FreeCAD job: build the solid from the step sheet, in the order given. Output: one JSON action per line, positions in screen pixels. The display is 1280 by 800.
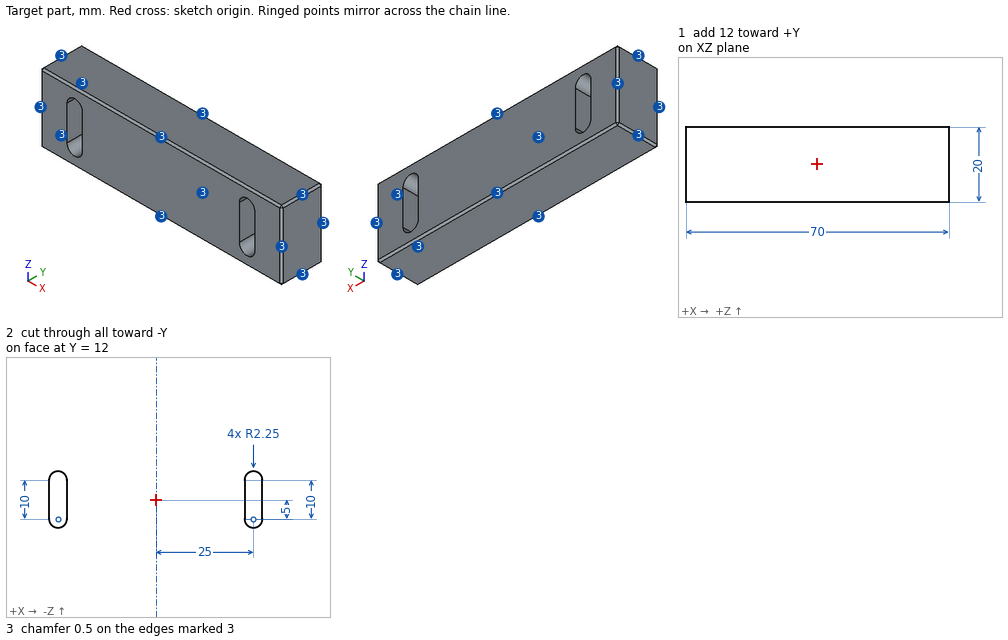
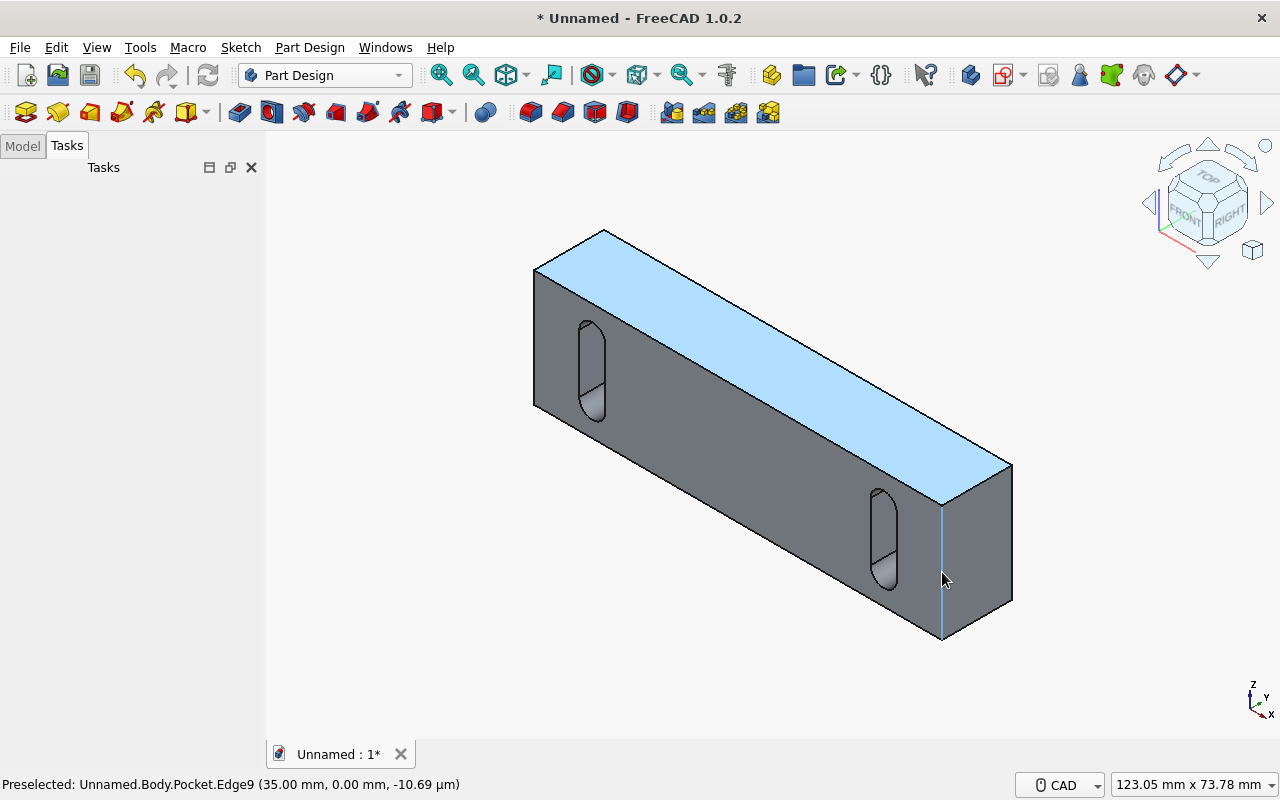
{"action": "key", "text": "2"}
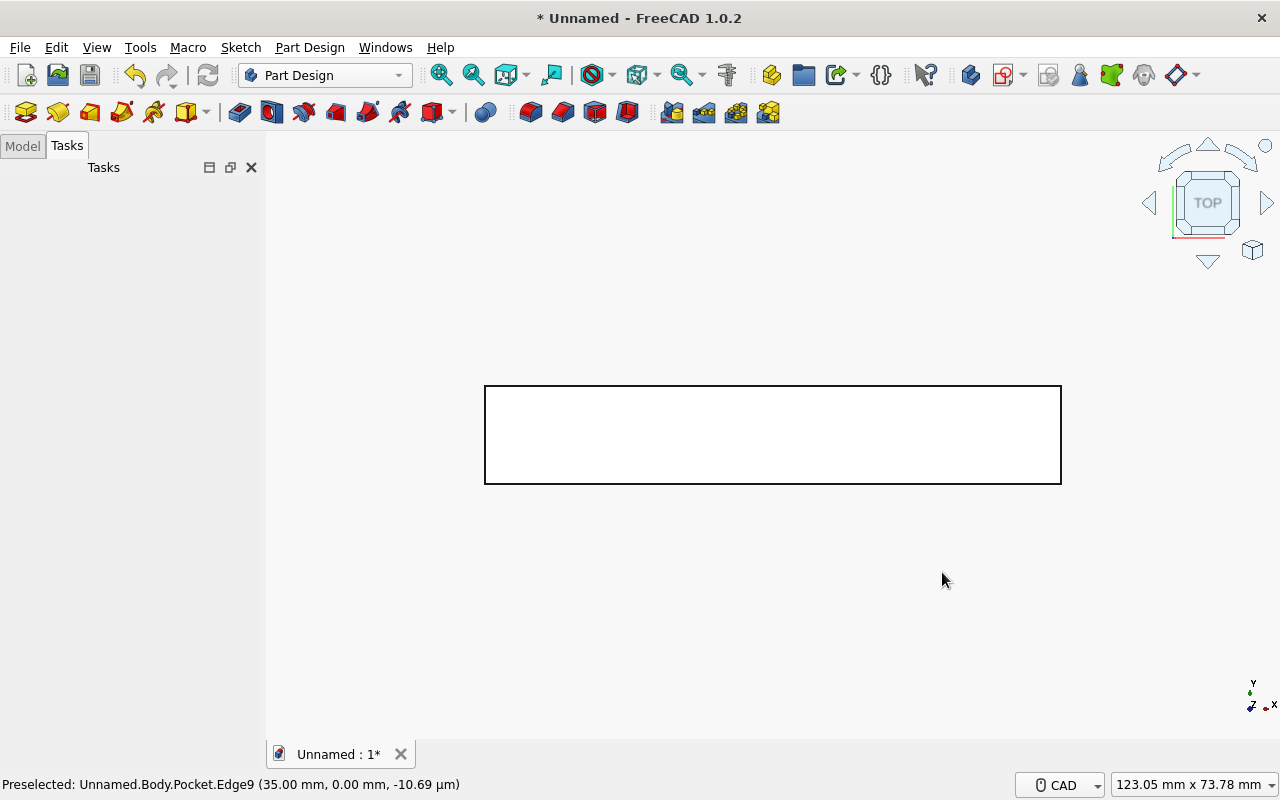
{"action": "key", "text": "1"}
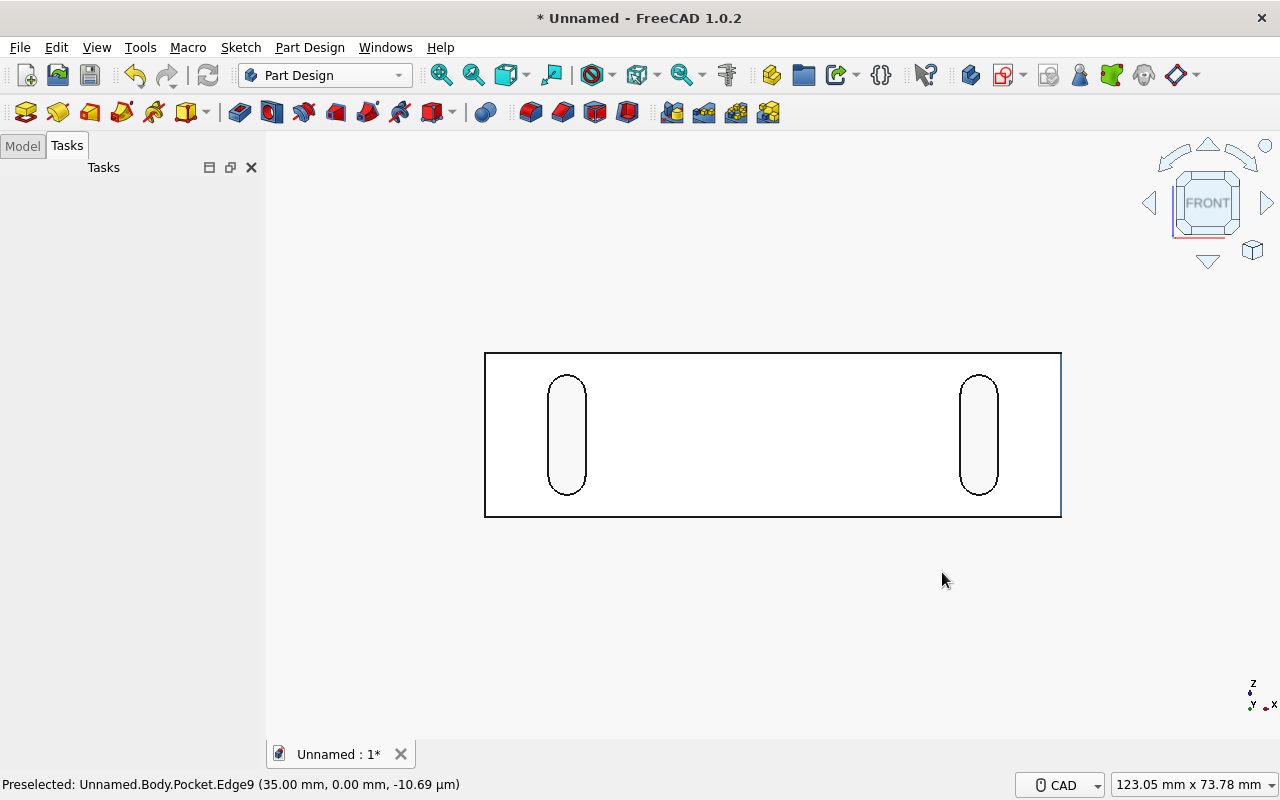
{"action": "key", "text": "3"}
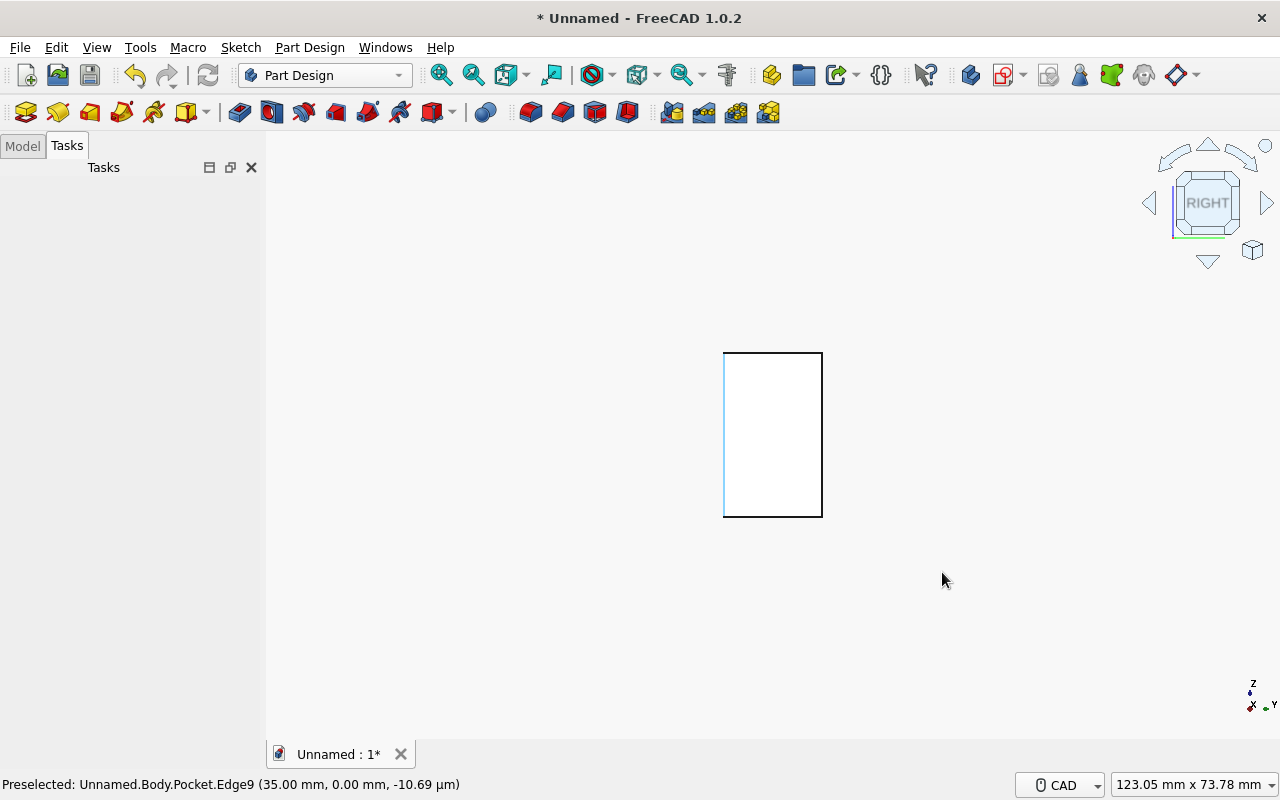
{"action": "key", "text": "v f"}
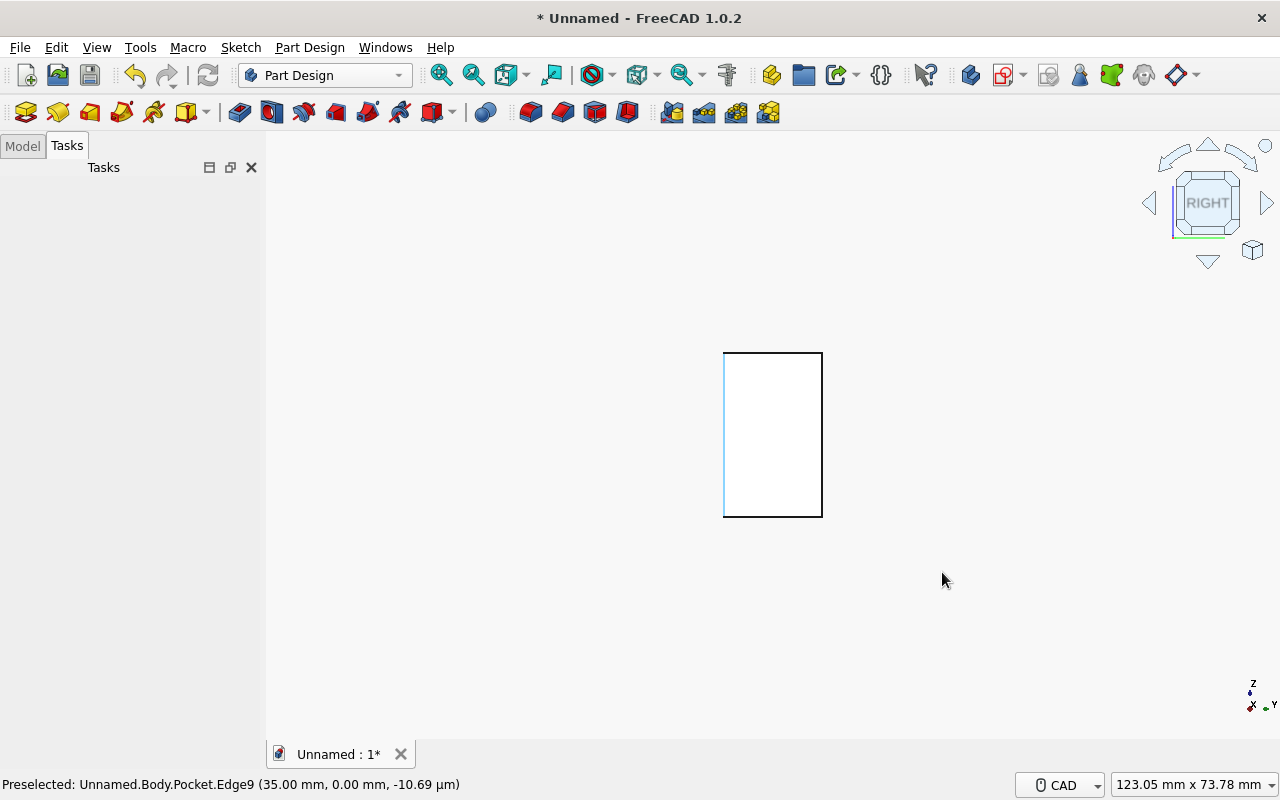
{"action": "left_click", "coordinate": [822, 434], "text": "ctrl"}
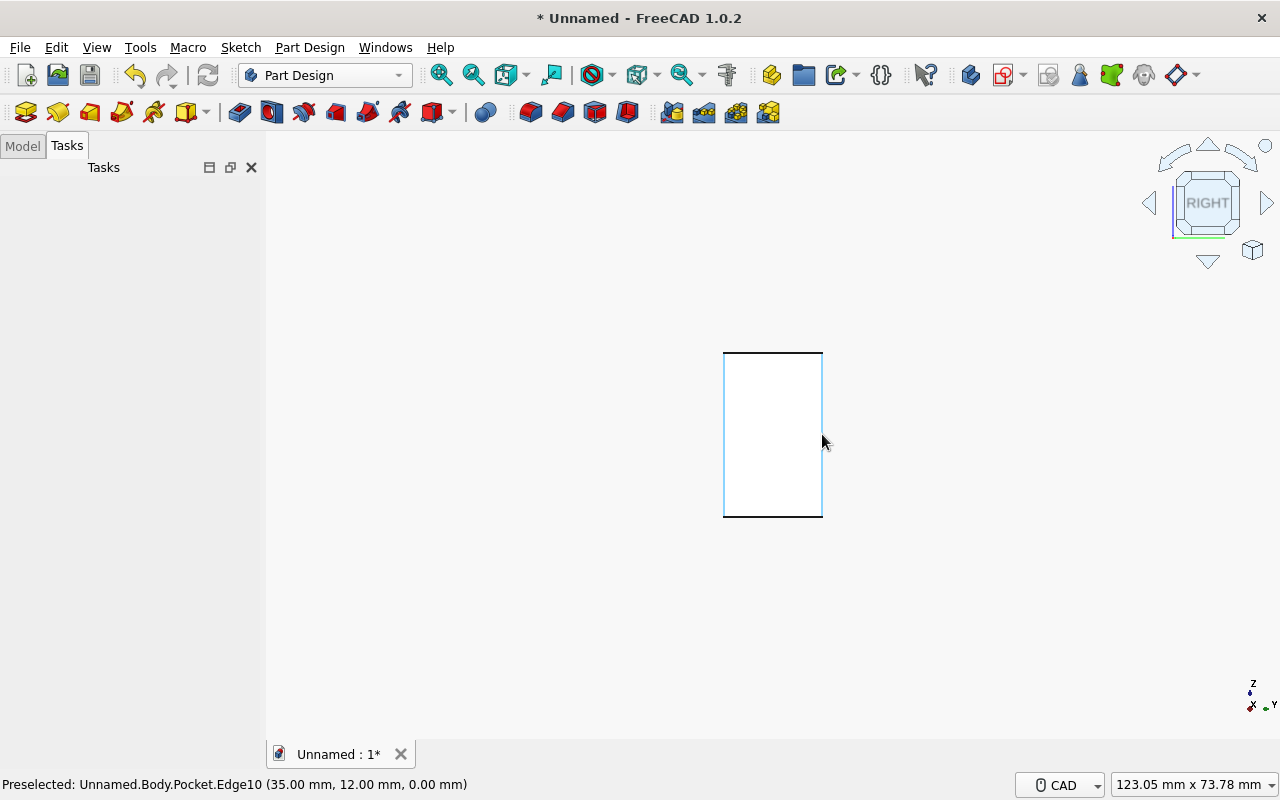
{"action": "key", "text": "5"}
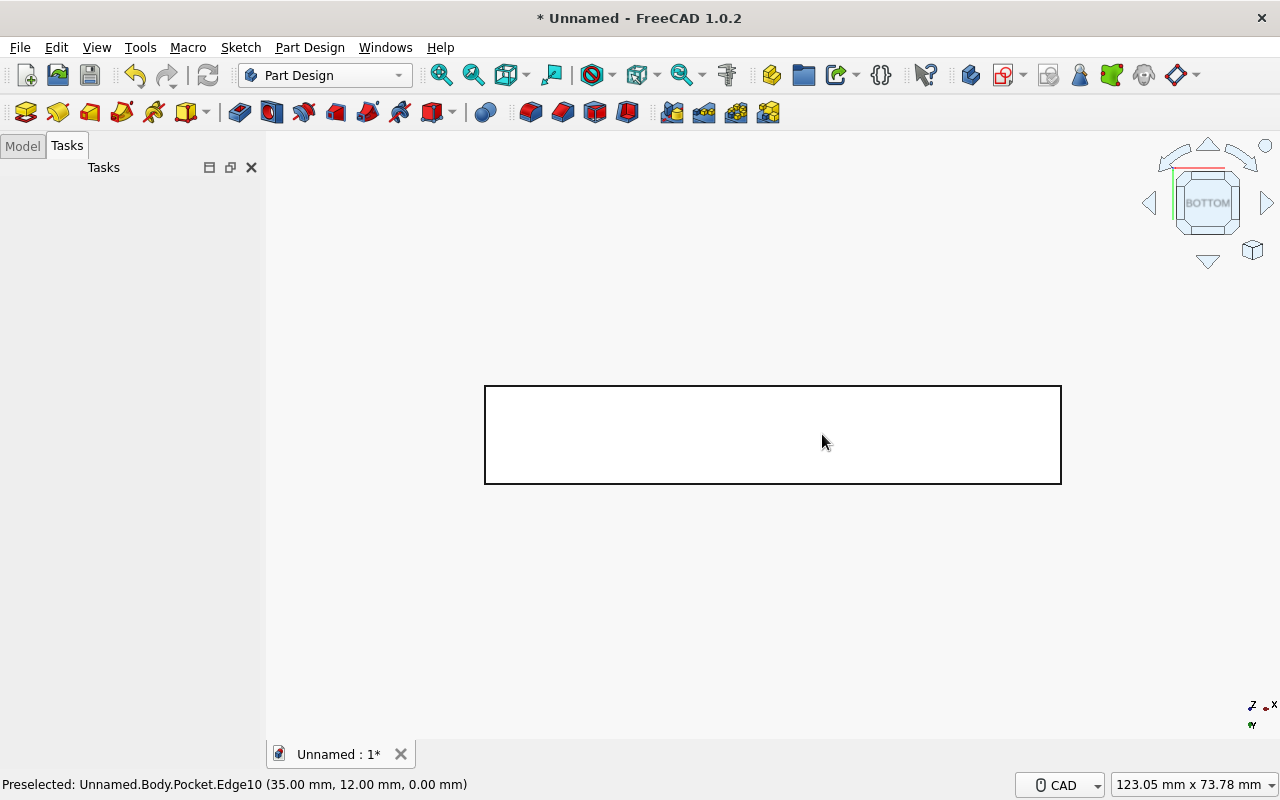
{"action": "left_click", "coordinate": [938, 434], "text": "ctrl"}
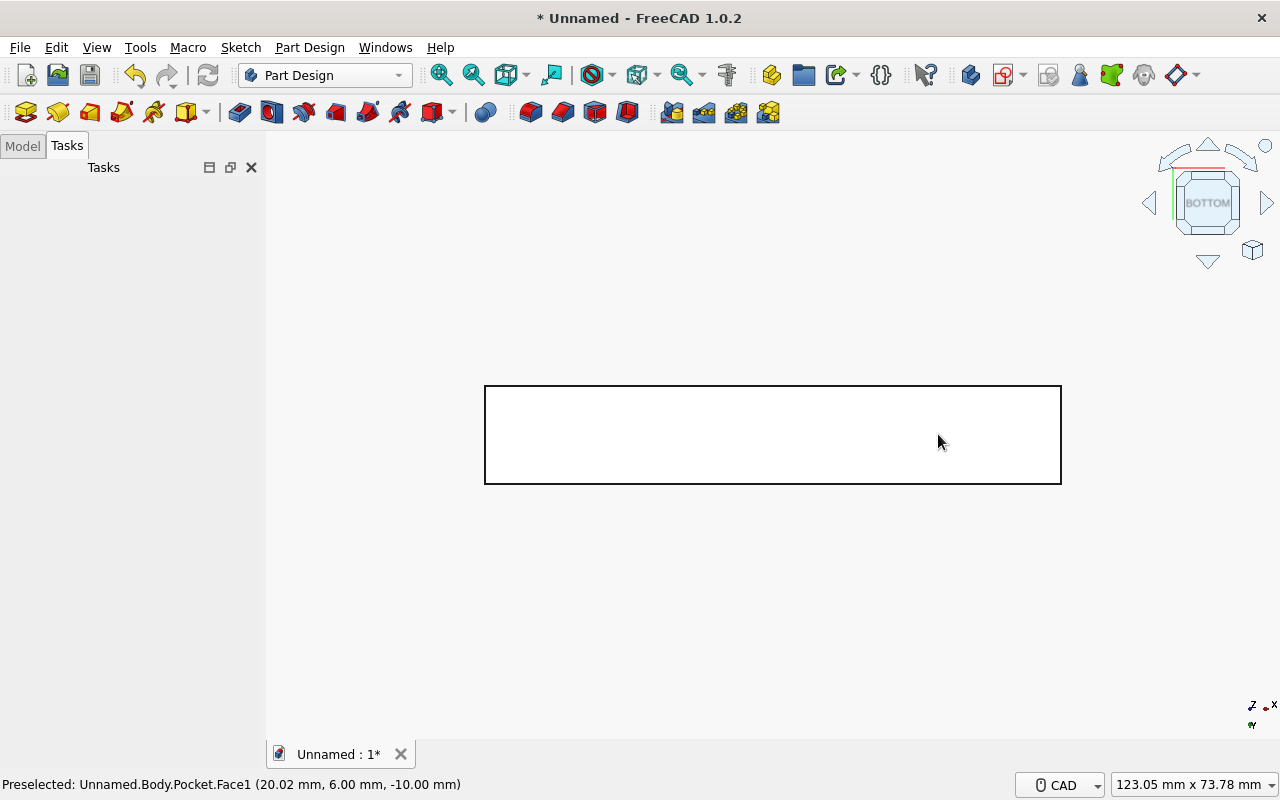
{"action": "key", "text": "4"}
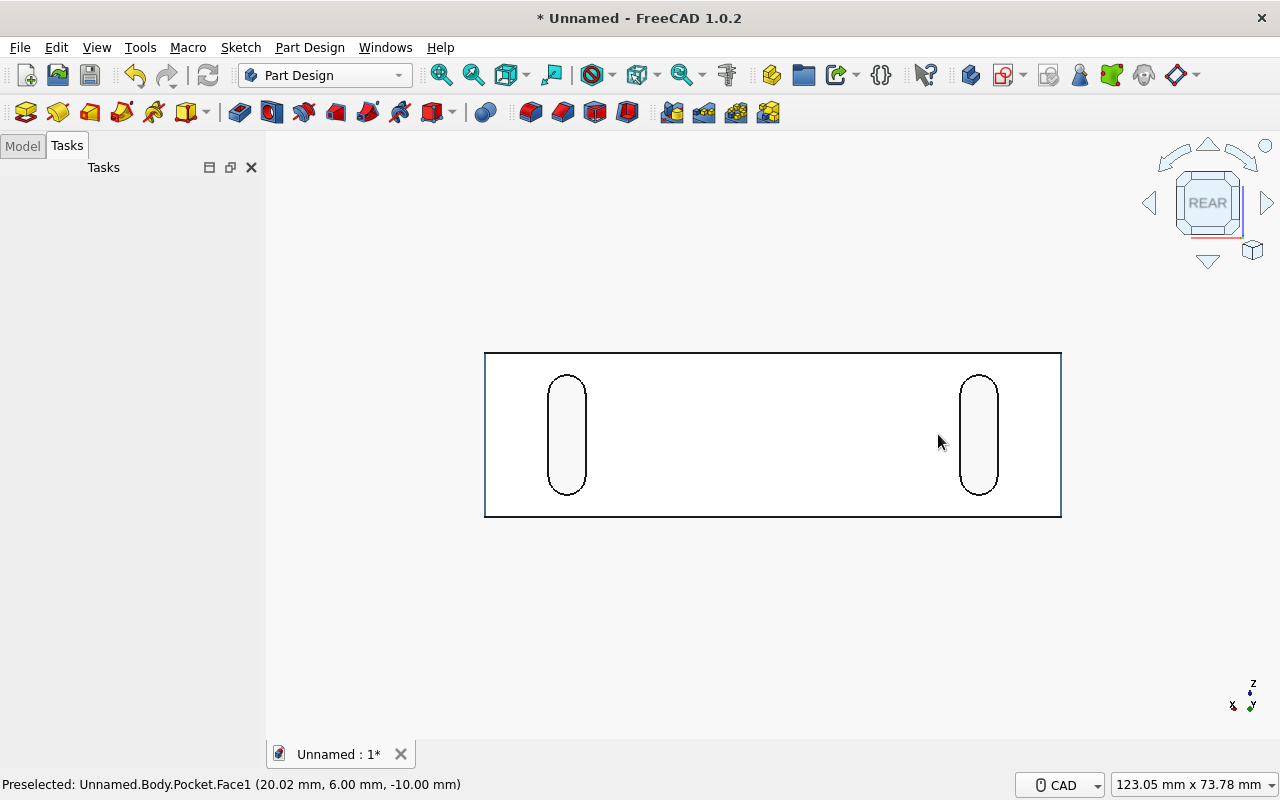
{"action": "key", "text": "6"}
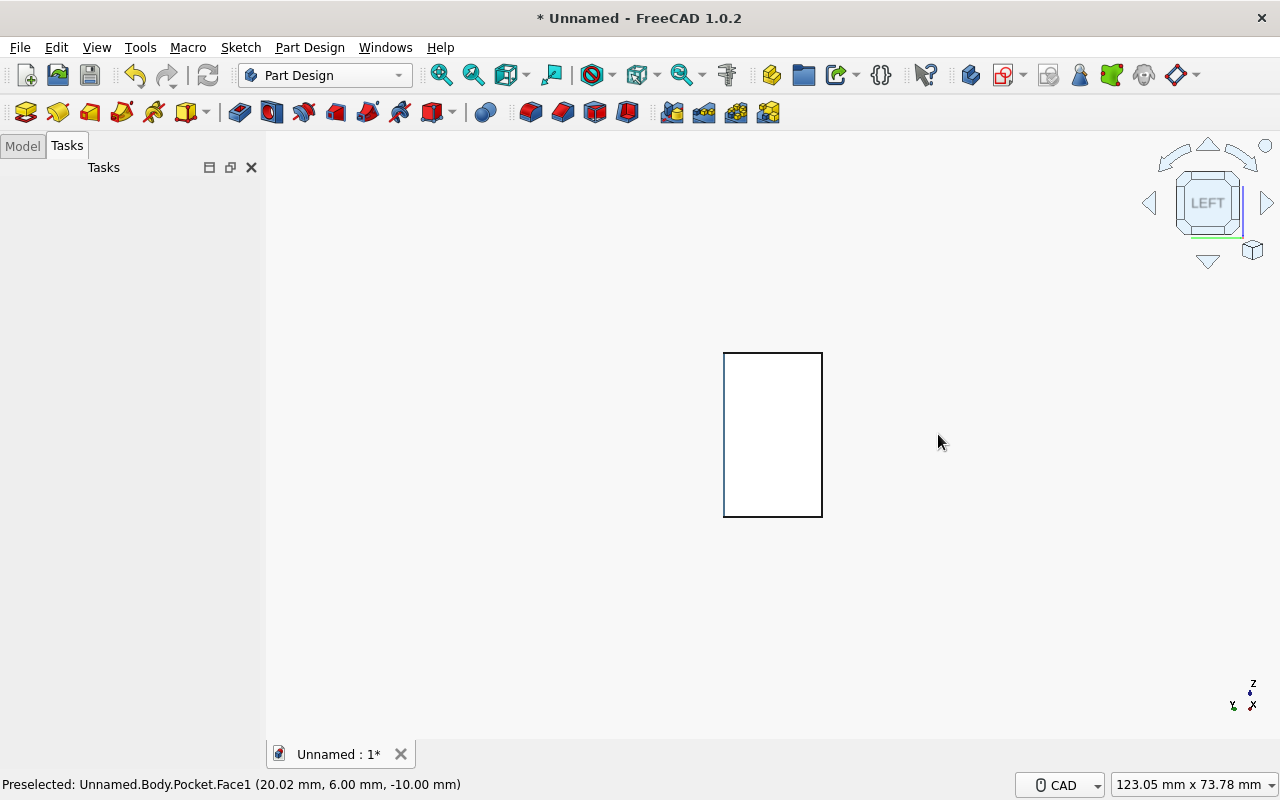
{"action": "key", "text": "v f"}